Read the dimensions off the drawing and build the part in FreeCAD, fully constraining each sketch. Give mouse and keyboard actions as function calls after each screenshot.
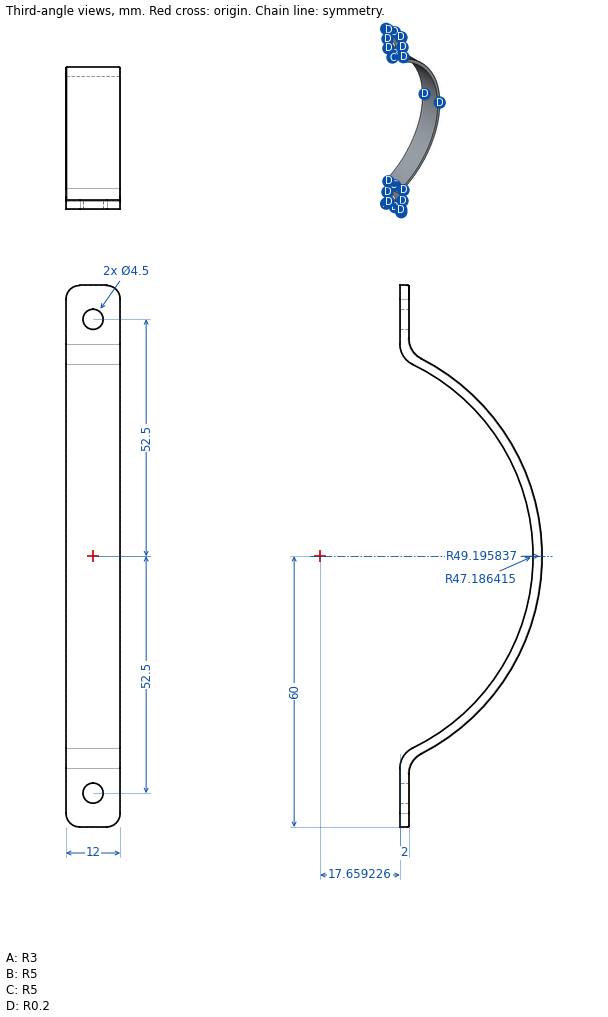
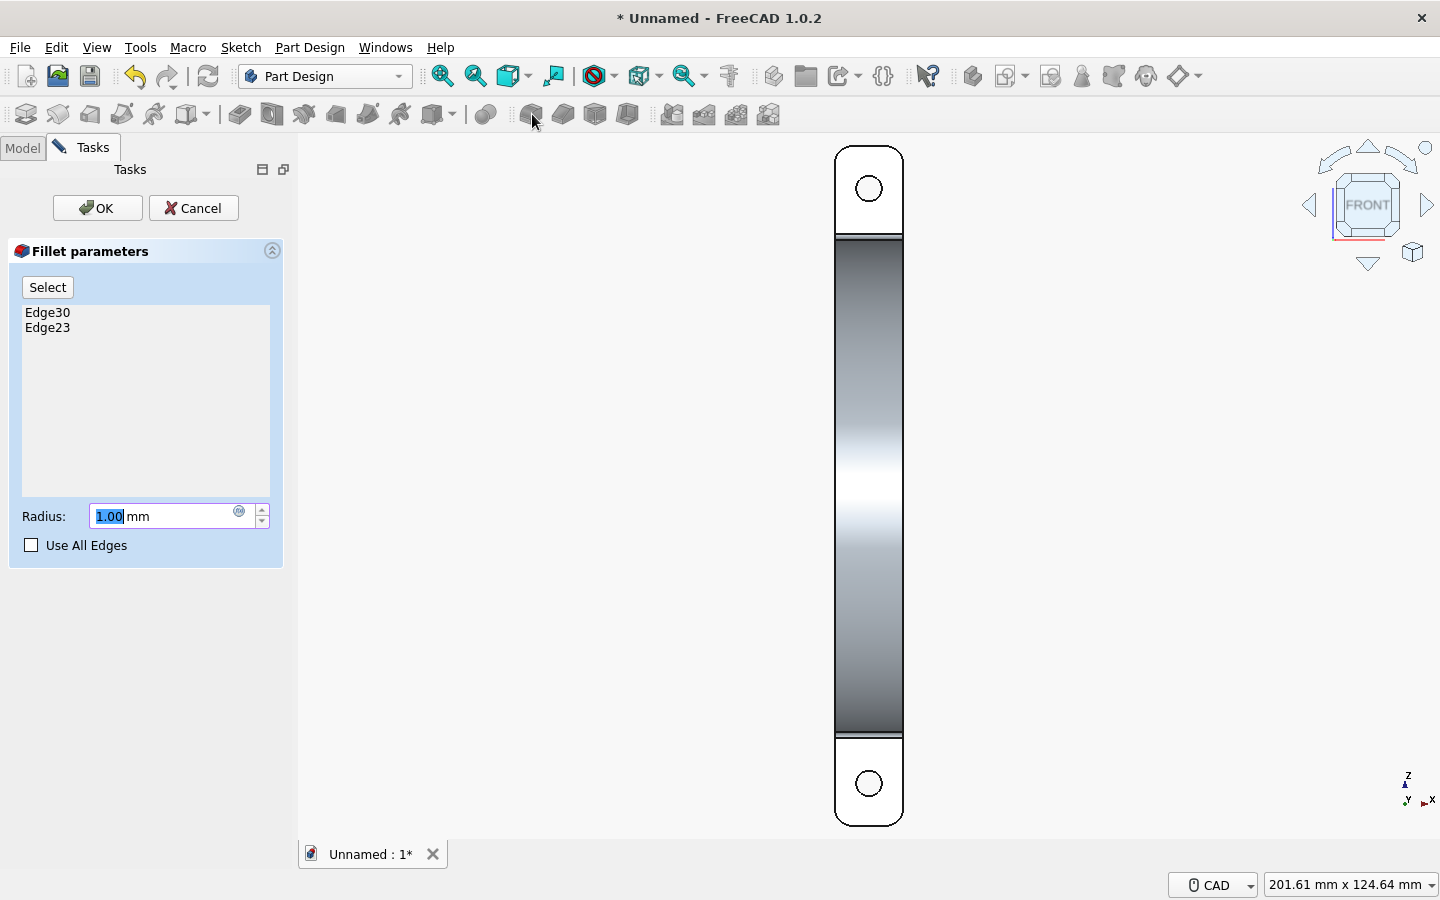
text(5)
key(Tab)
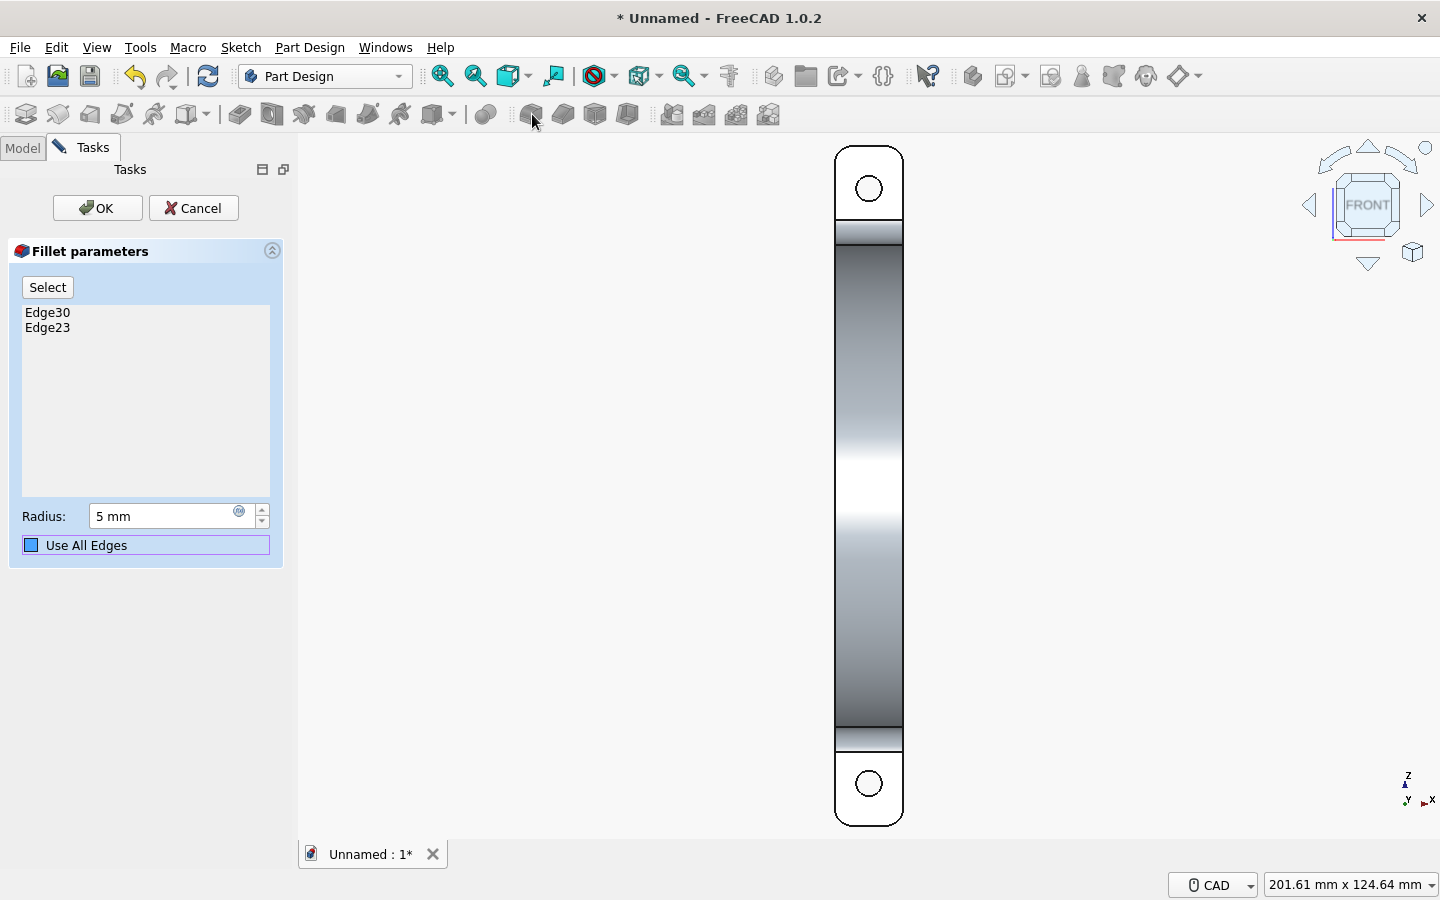
click(98, 208)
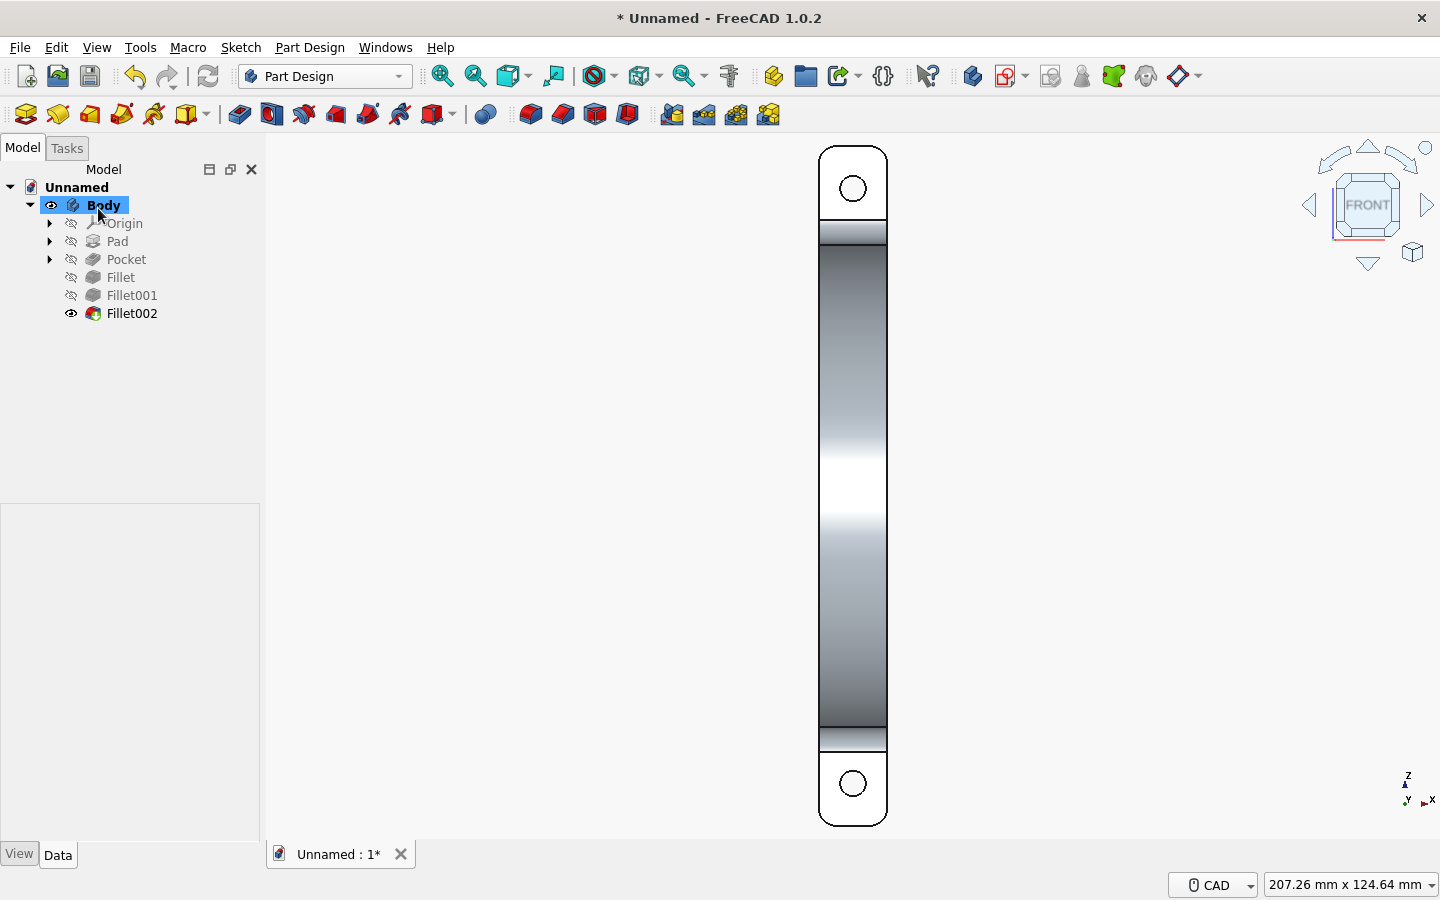
key(0)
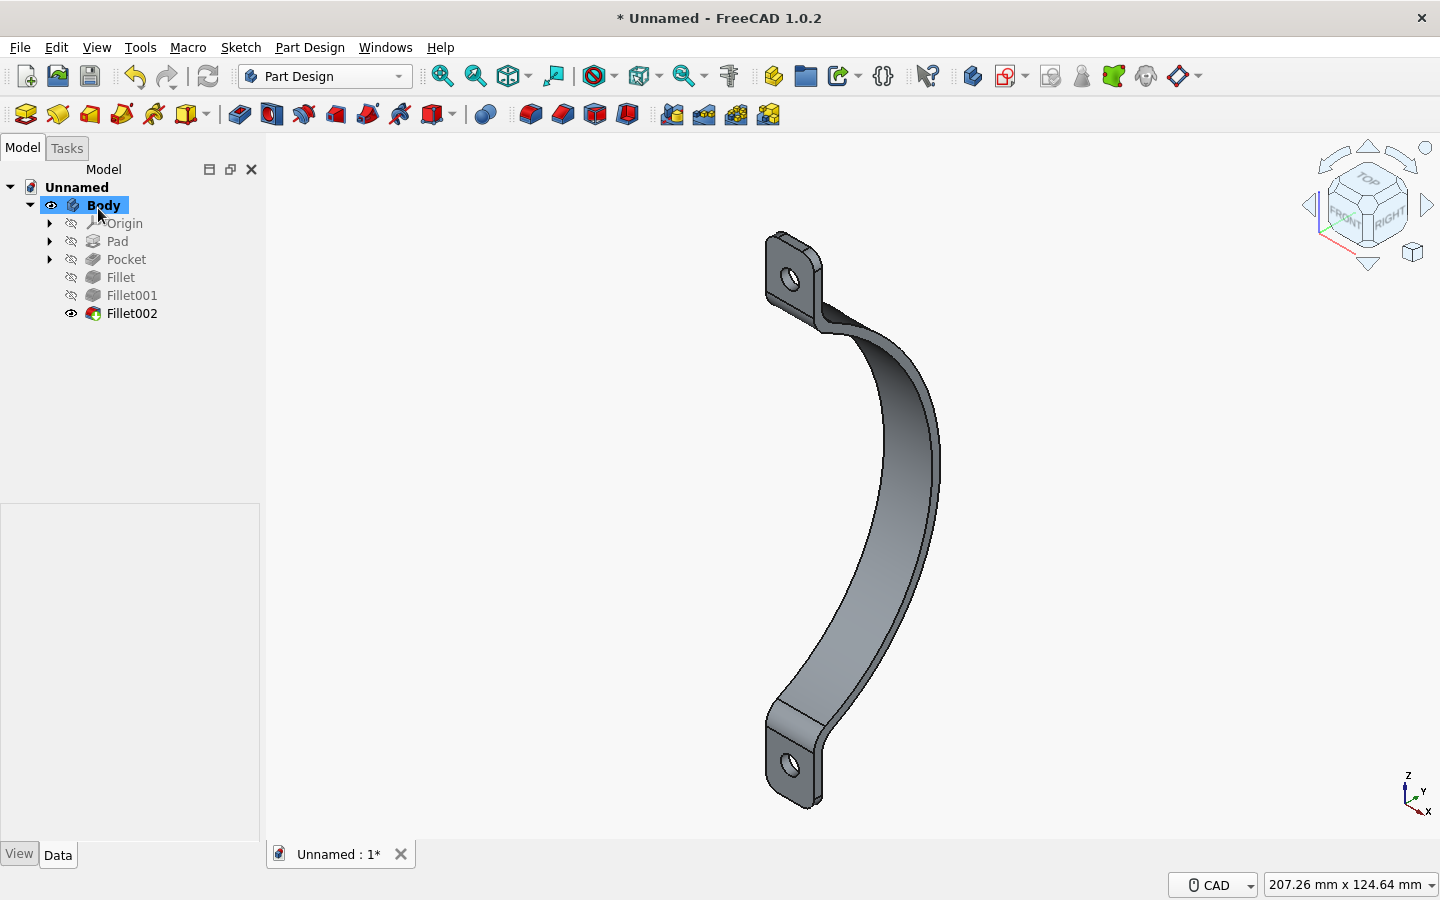
click(821, 260)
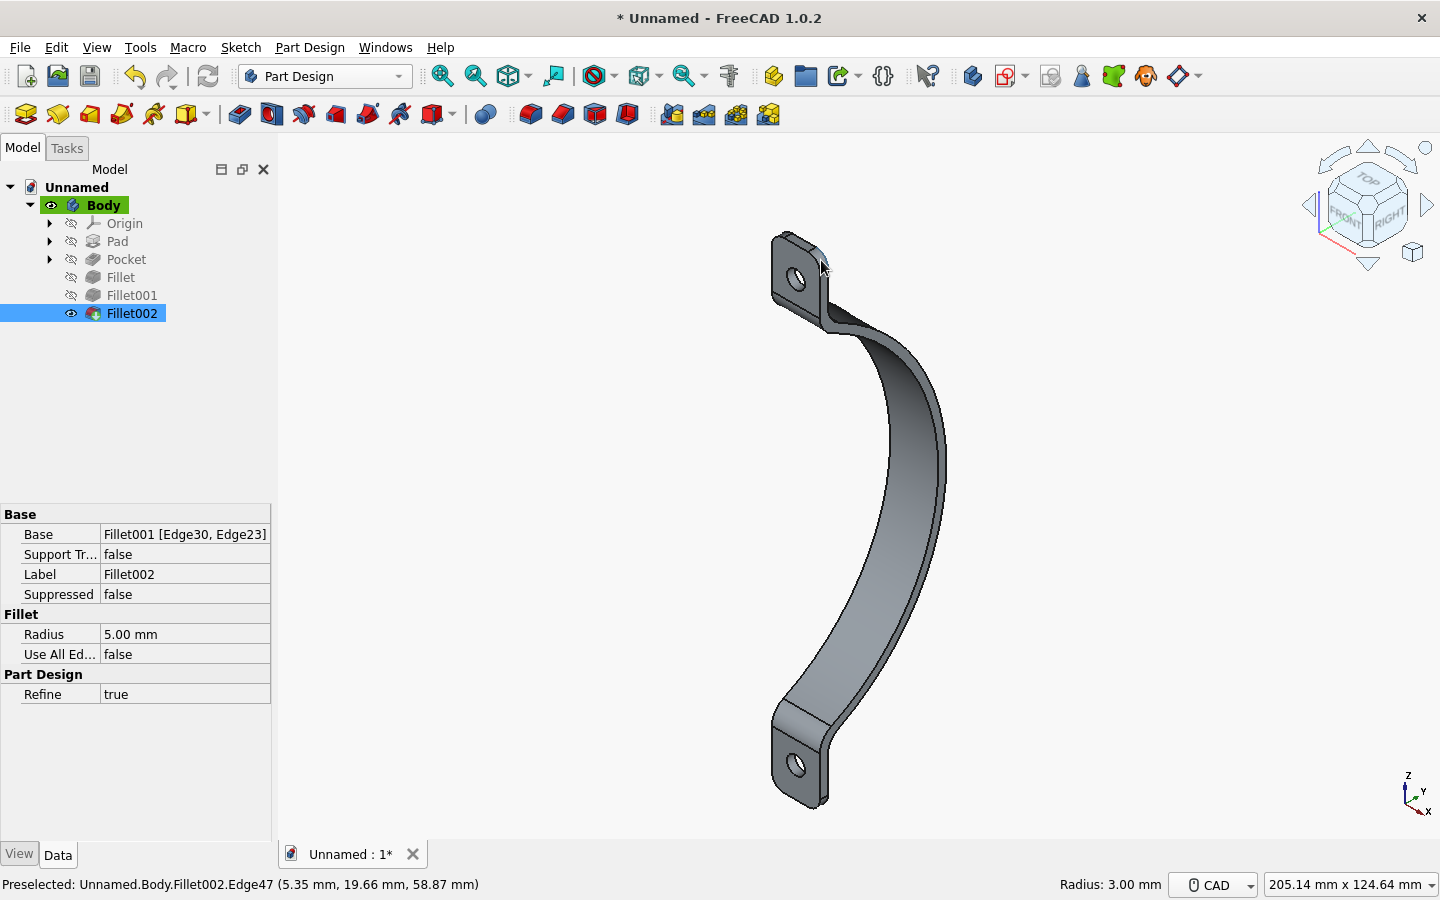
click(882, 331, ctrl)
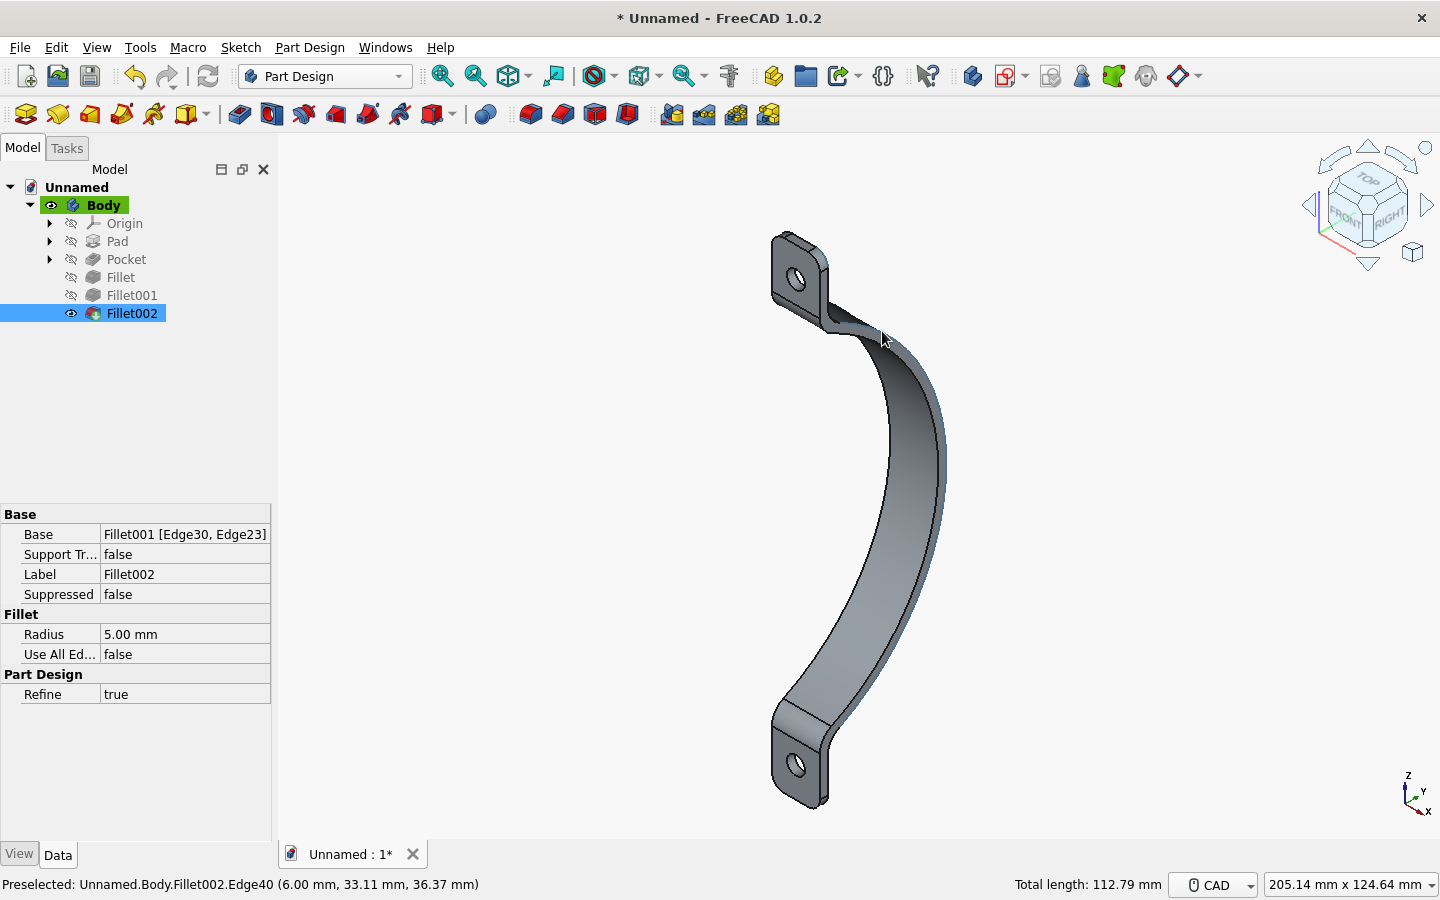
click(837, 321, ctrl)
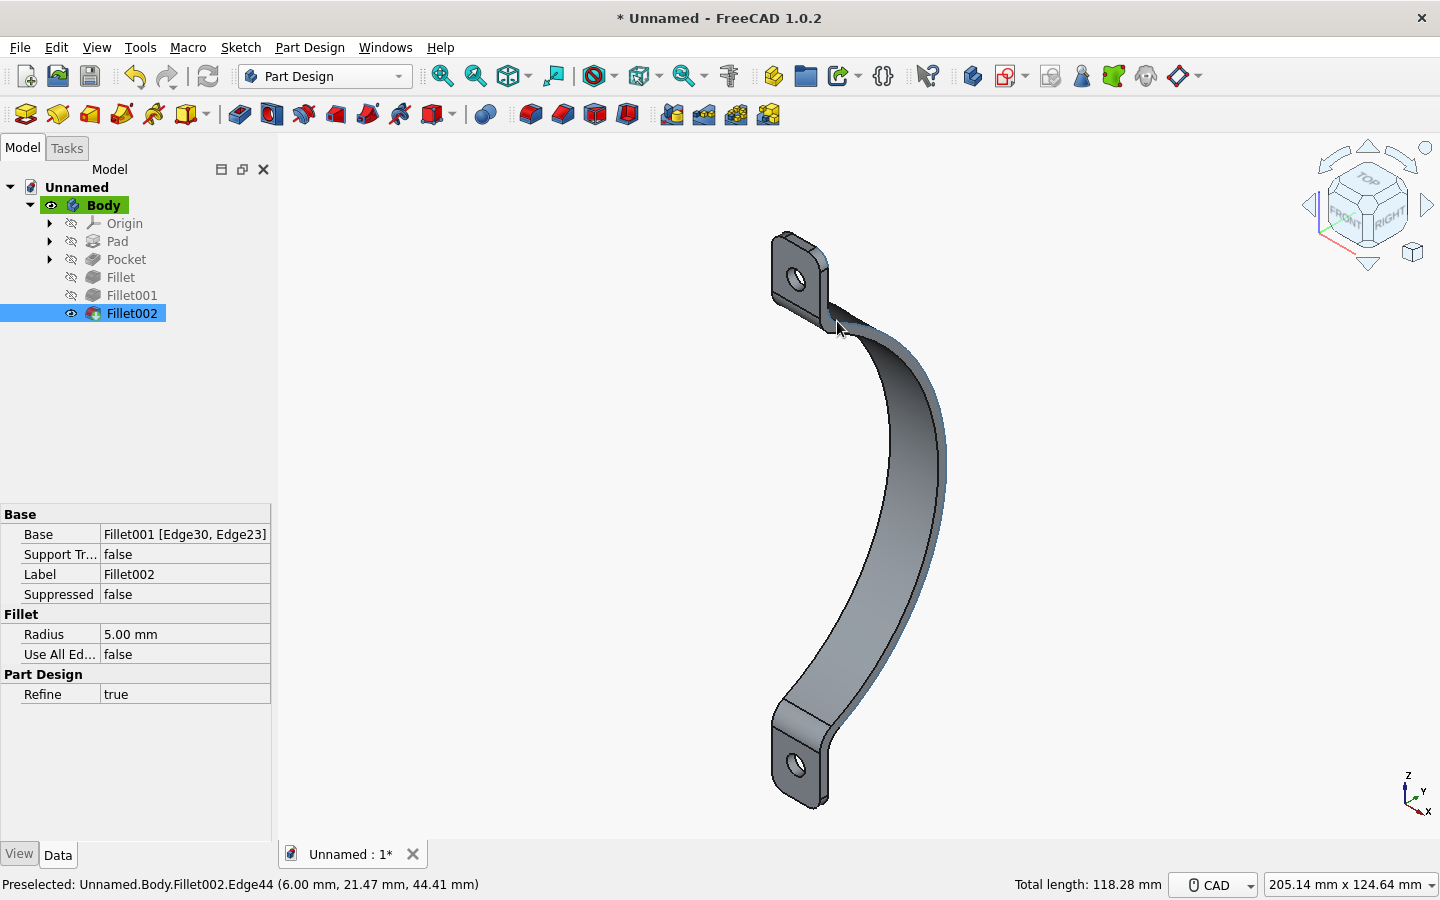
key(2)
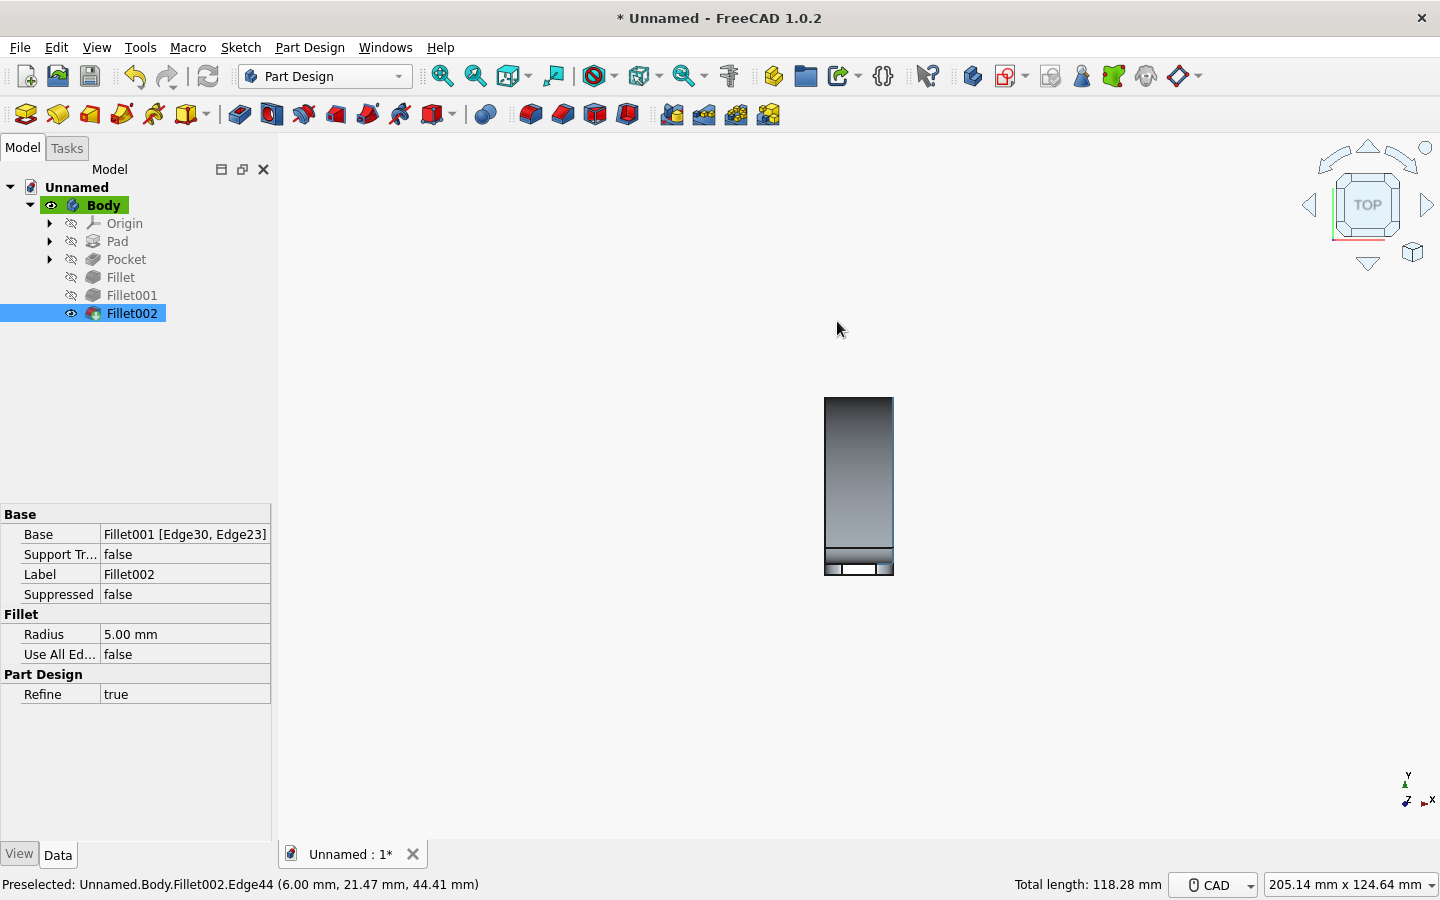
click(444, 76)